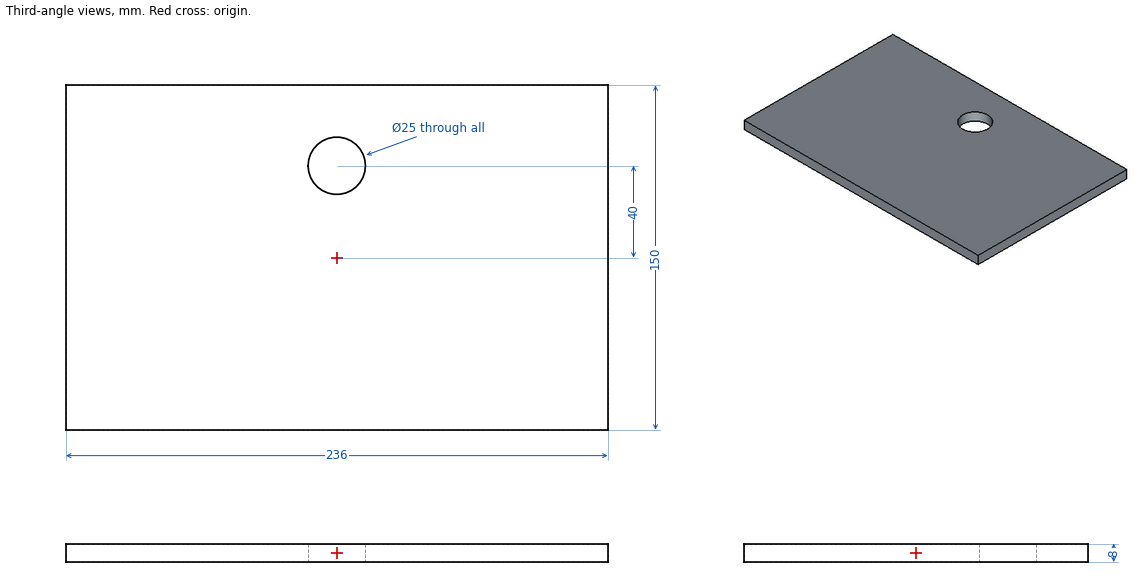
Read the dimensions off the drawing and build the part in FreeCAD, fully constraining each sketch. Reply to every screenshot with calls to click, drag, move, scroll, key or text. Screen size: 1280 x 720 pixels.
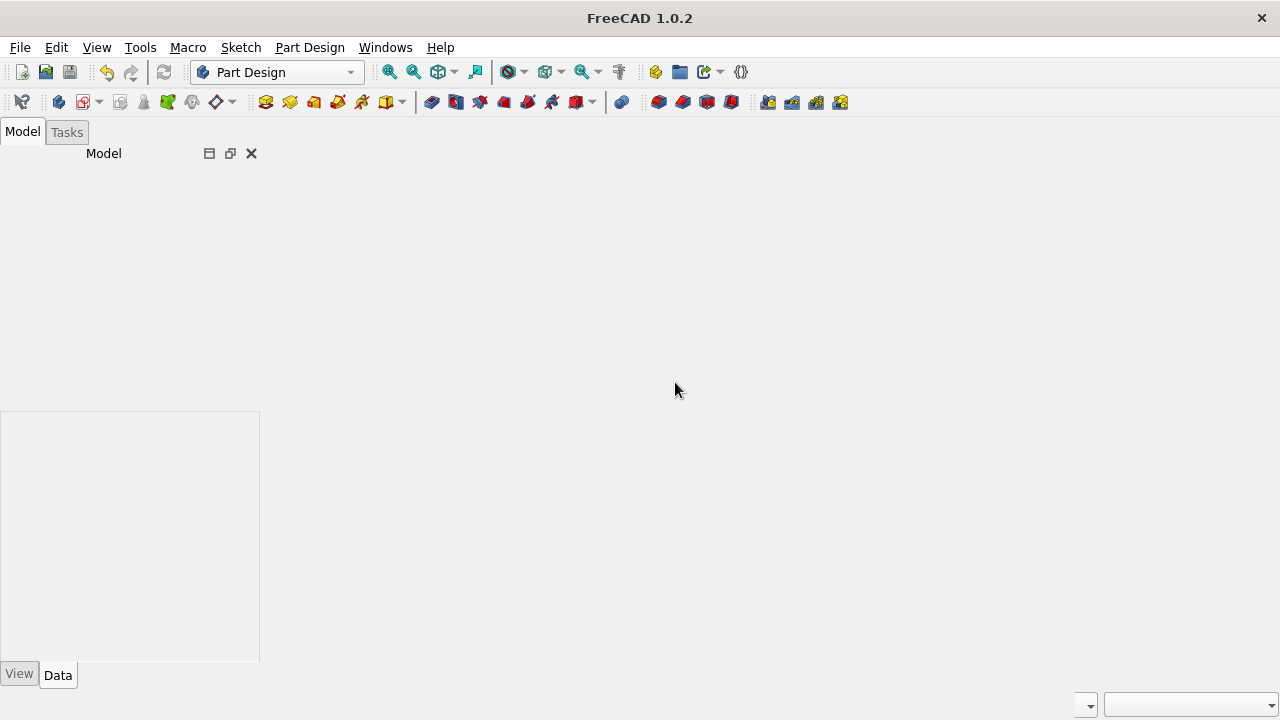
click(22, 72)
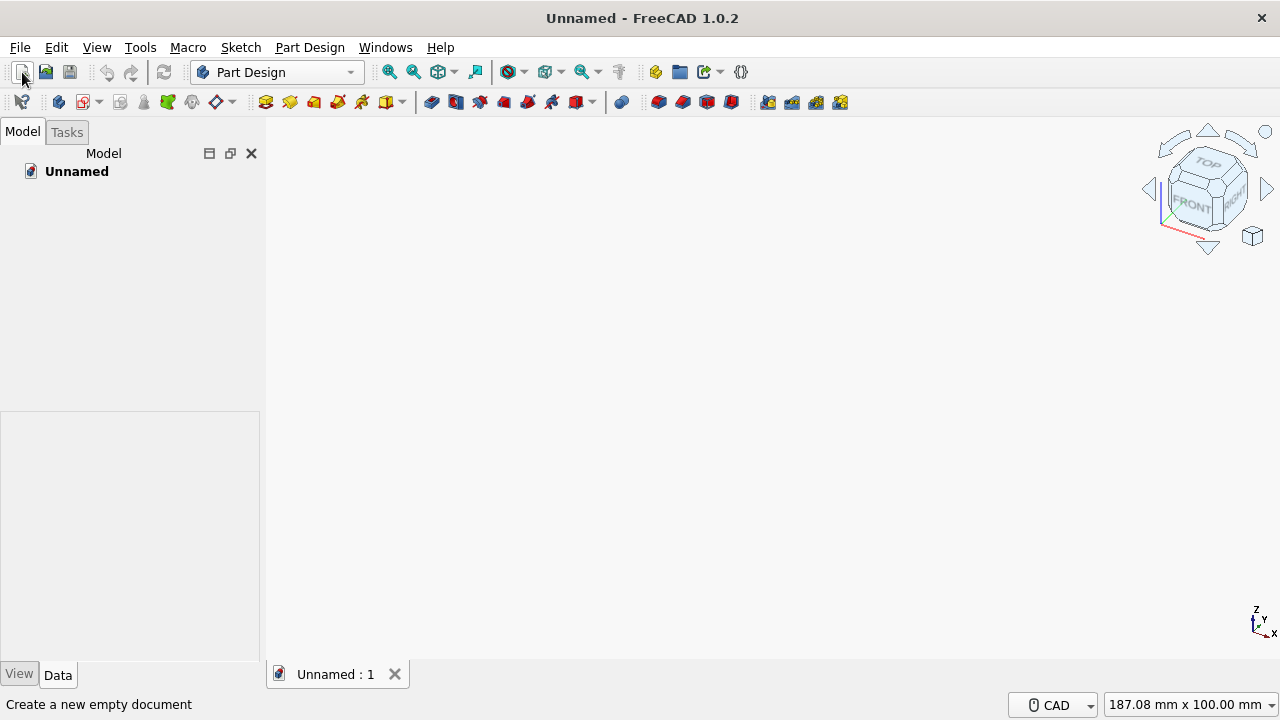
click(84, 102)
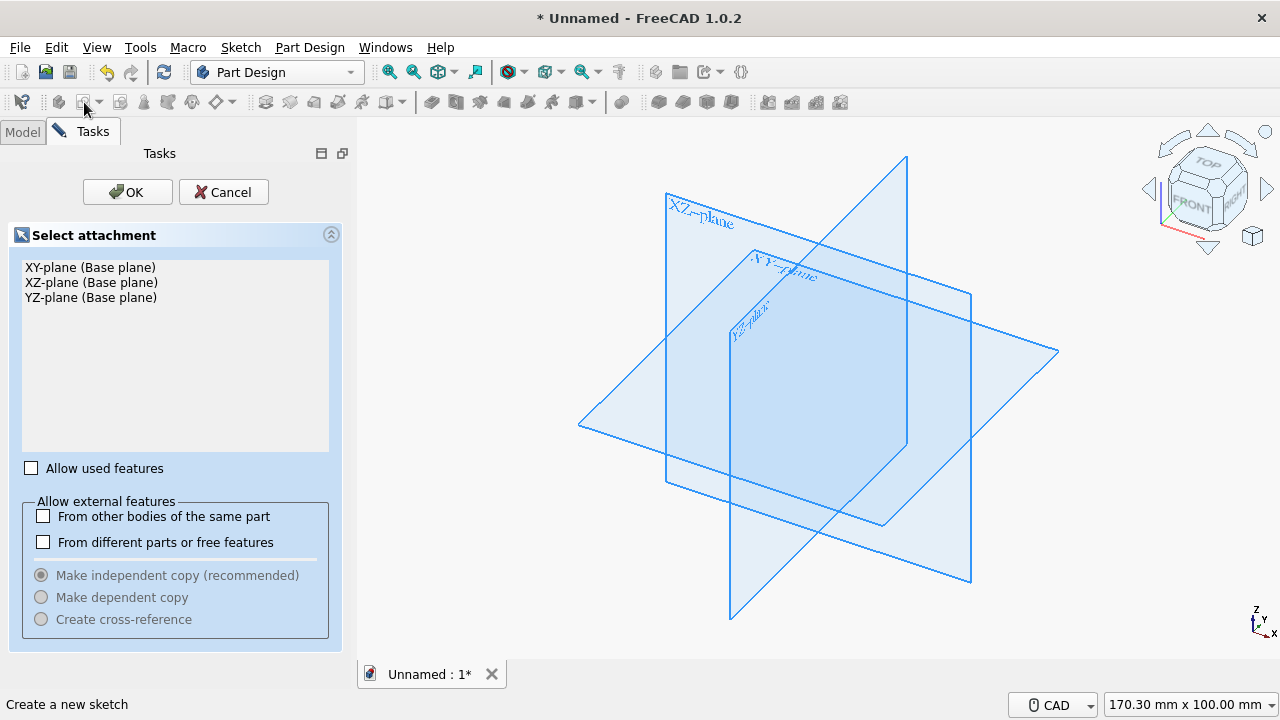
click(82, 268)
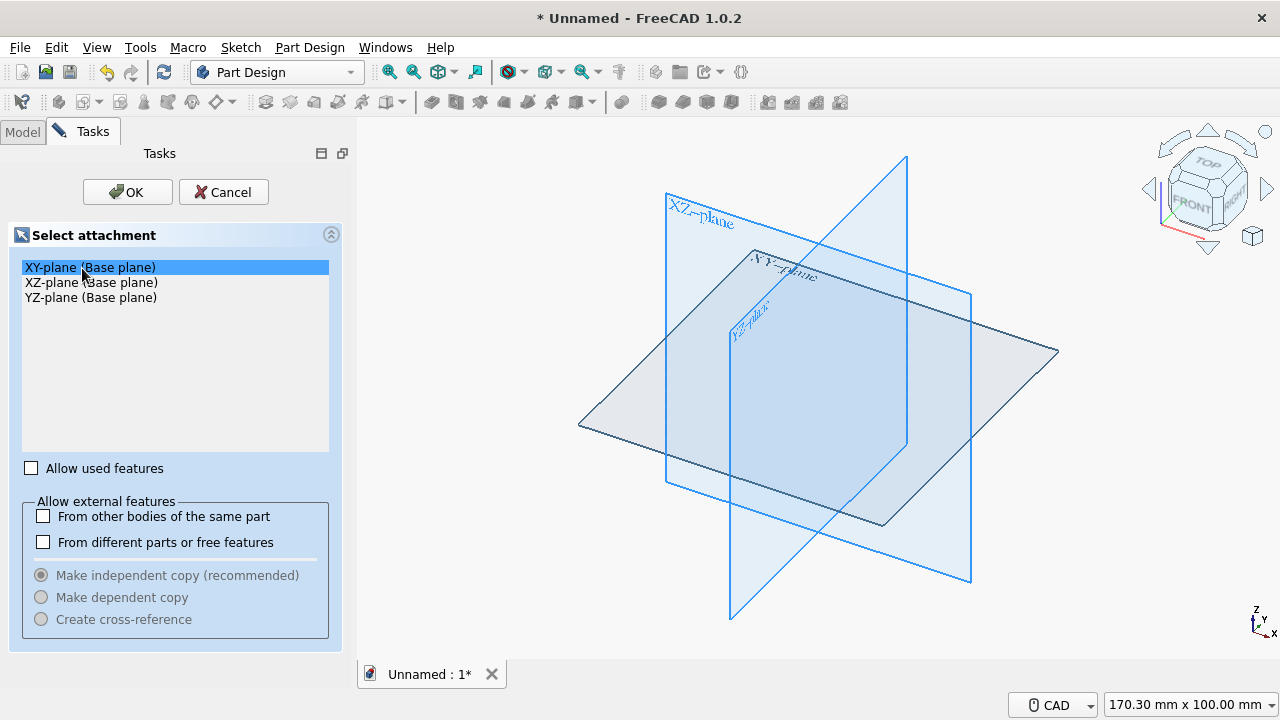
click(128, 192)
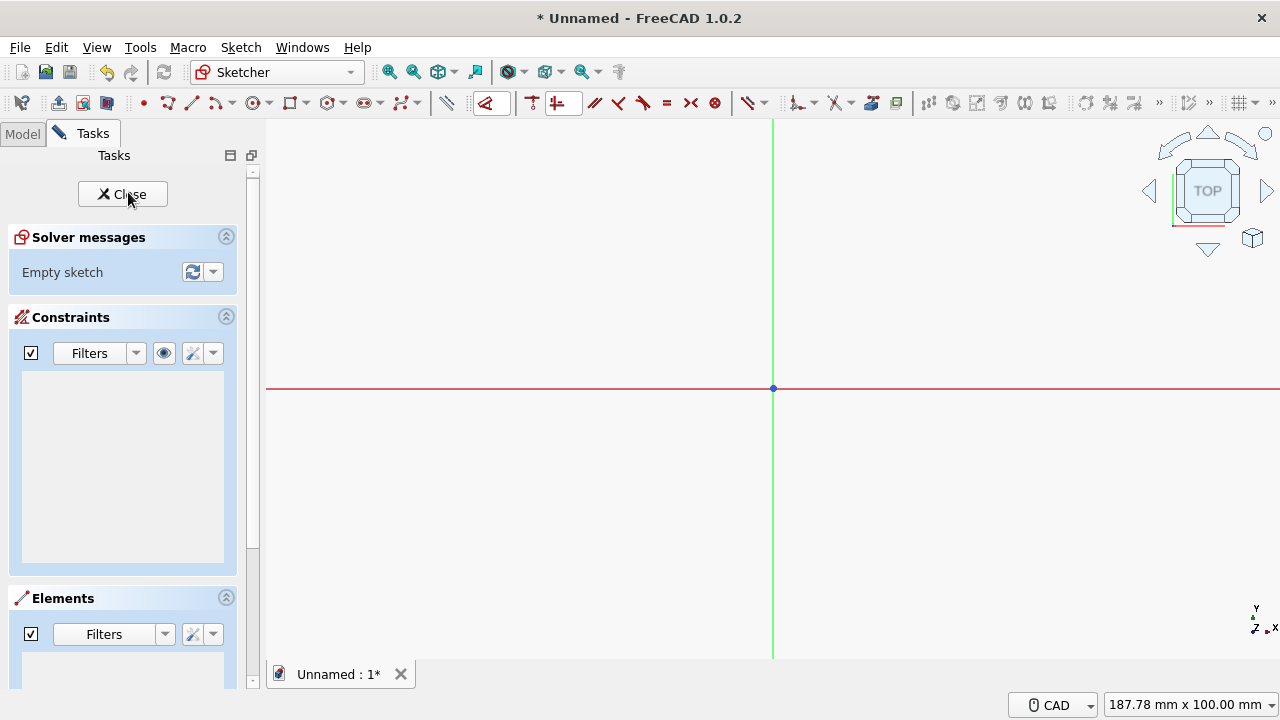
scroll(649, 389, down, 4)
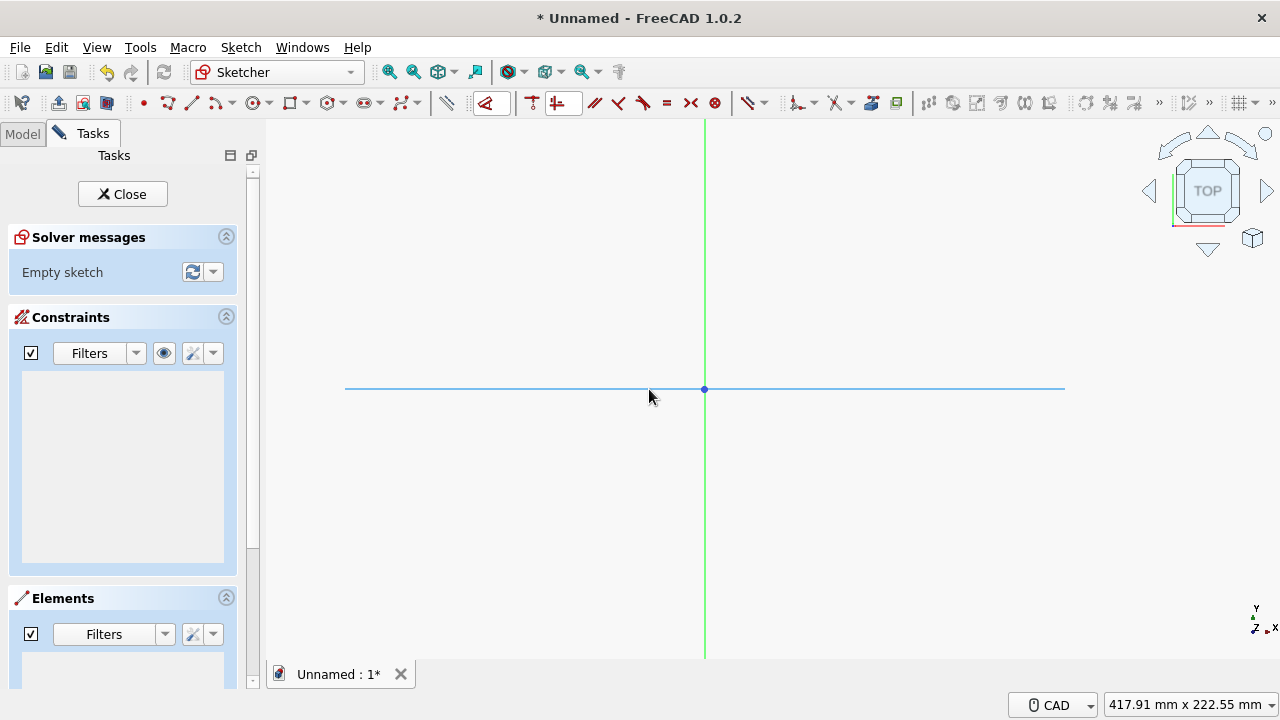
key(g)
key(v)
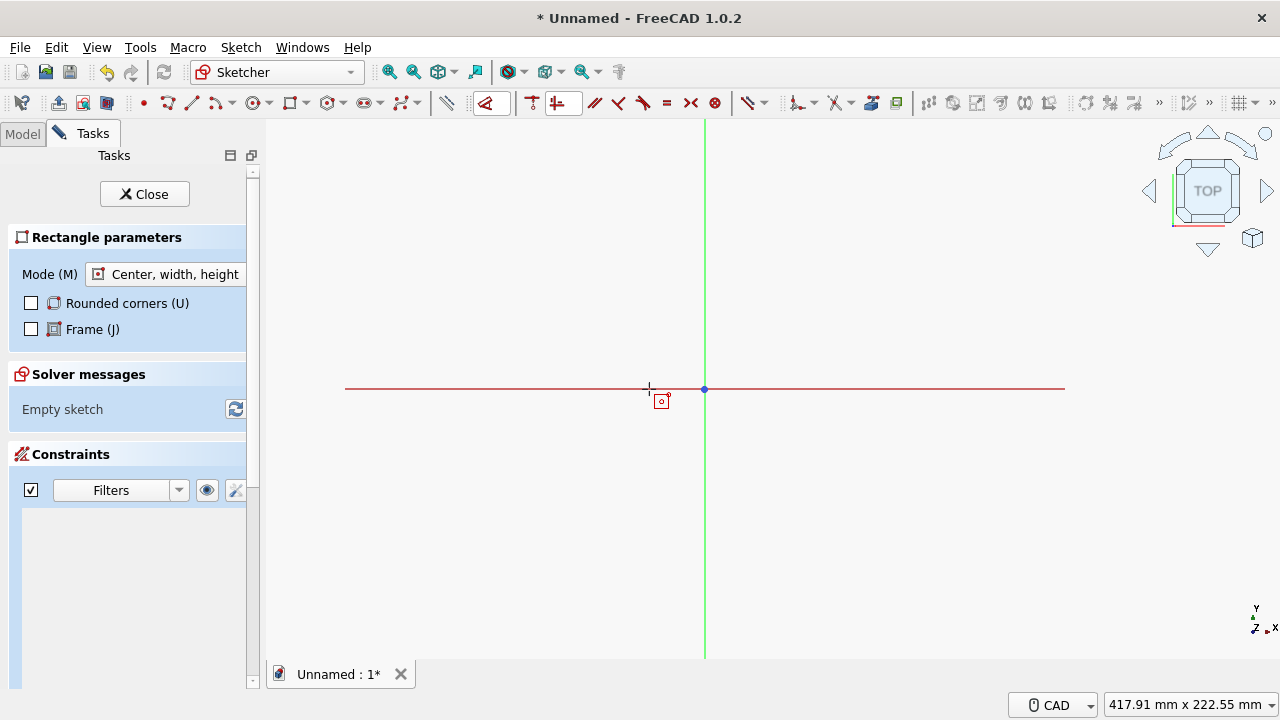
click(705, 389)
click(991, 207)
key(Escape)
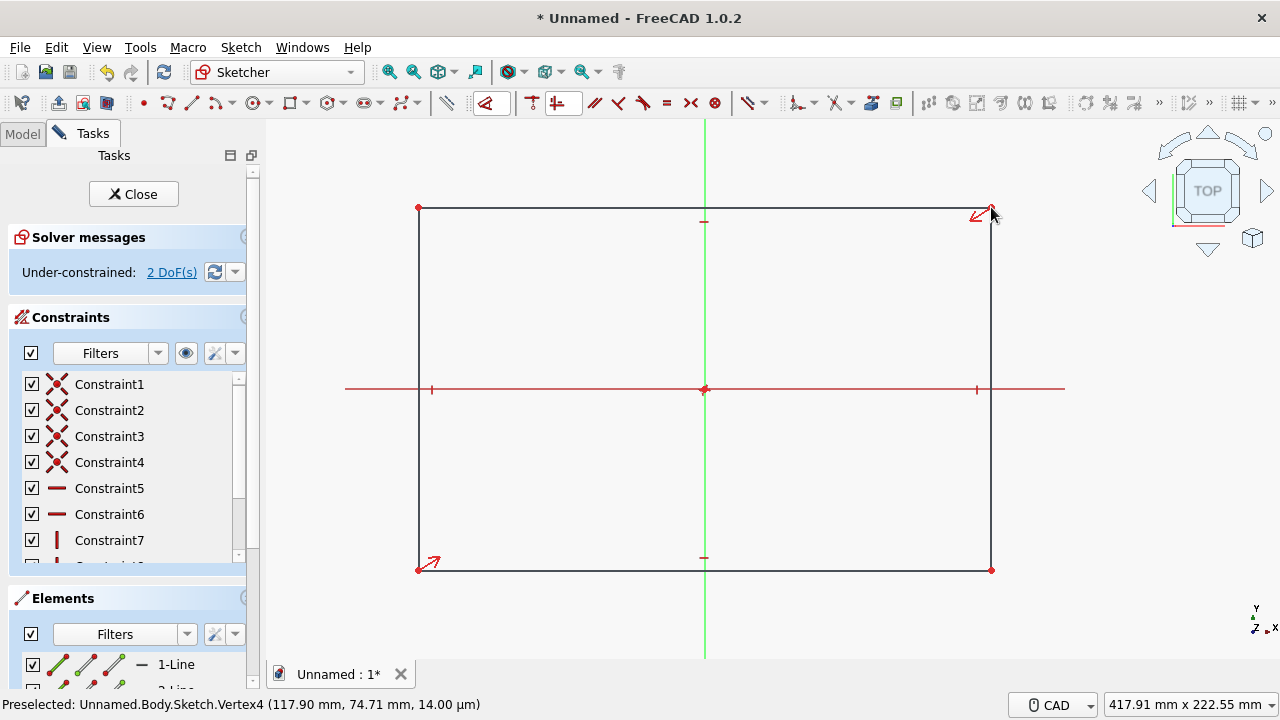
key(d)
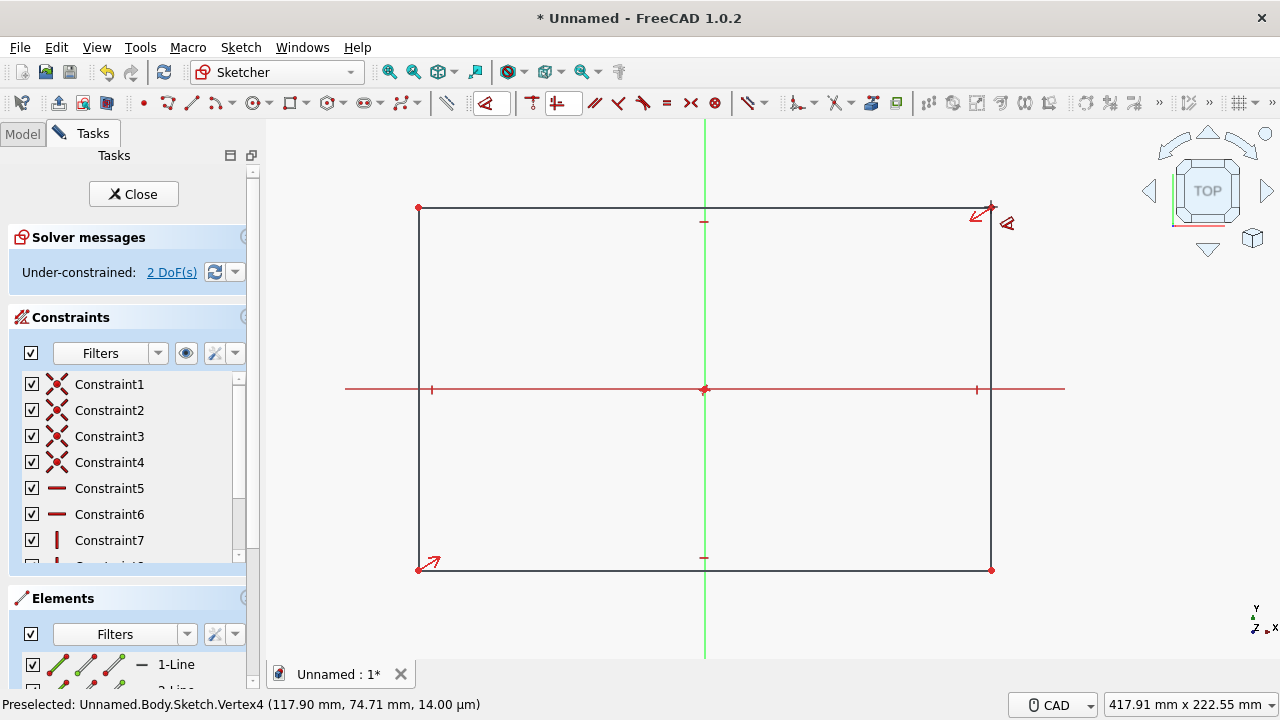
click(590, 571)
click(573, 605)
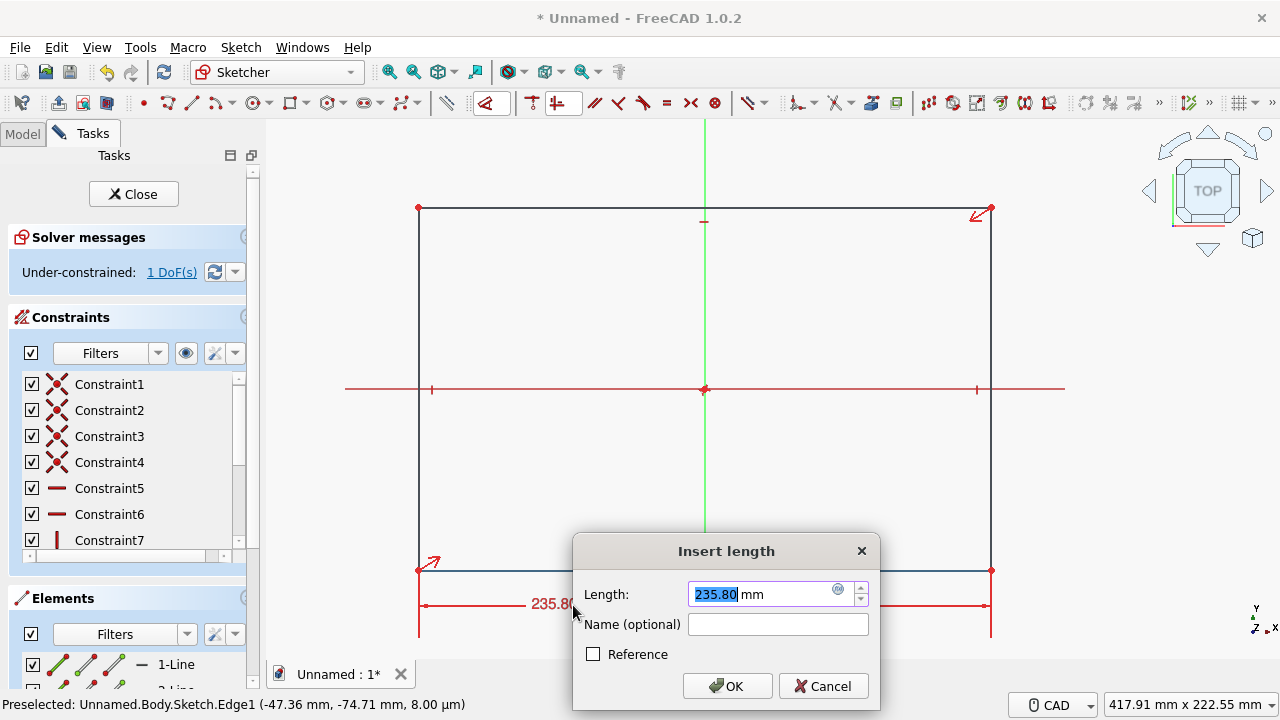
text(236)
key(Return)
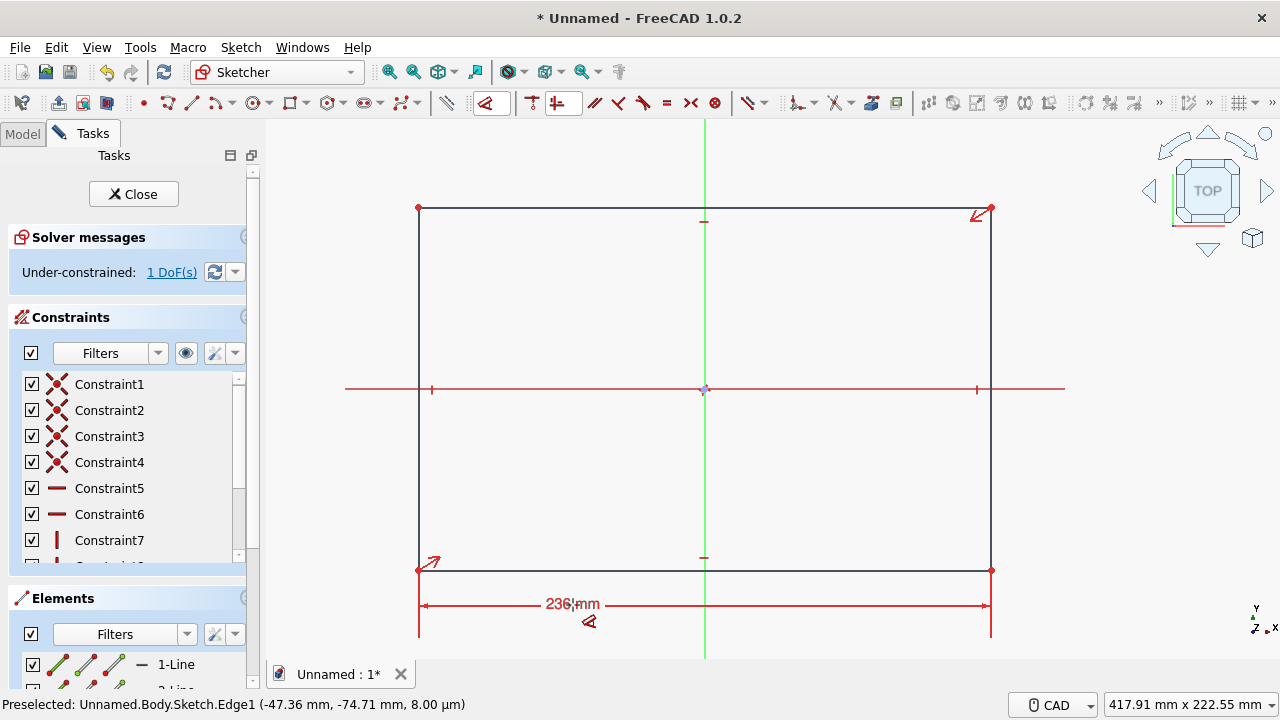
click(991, 462)
click(1025, 306)